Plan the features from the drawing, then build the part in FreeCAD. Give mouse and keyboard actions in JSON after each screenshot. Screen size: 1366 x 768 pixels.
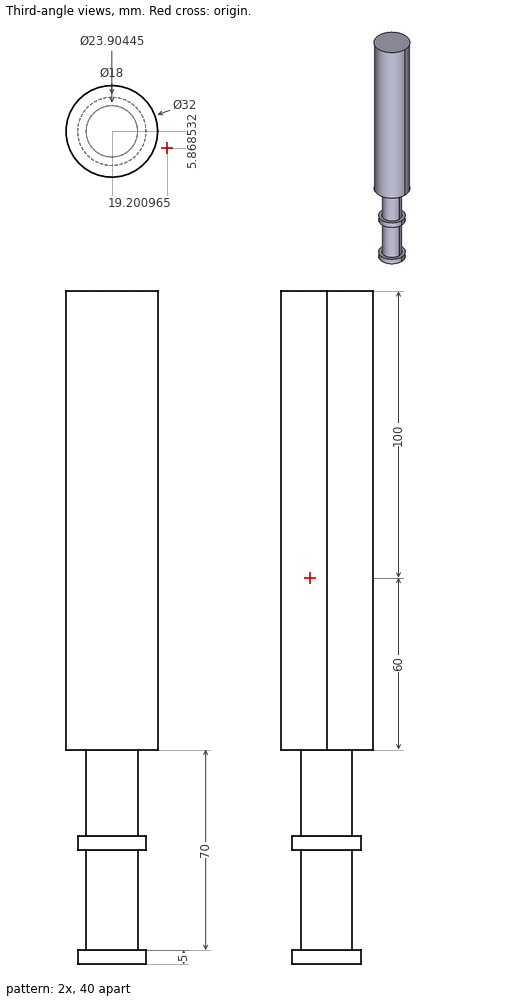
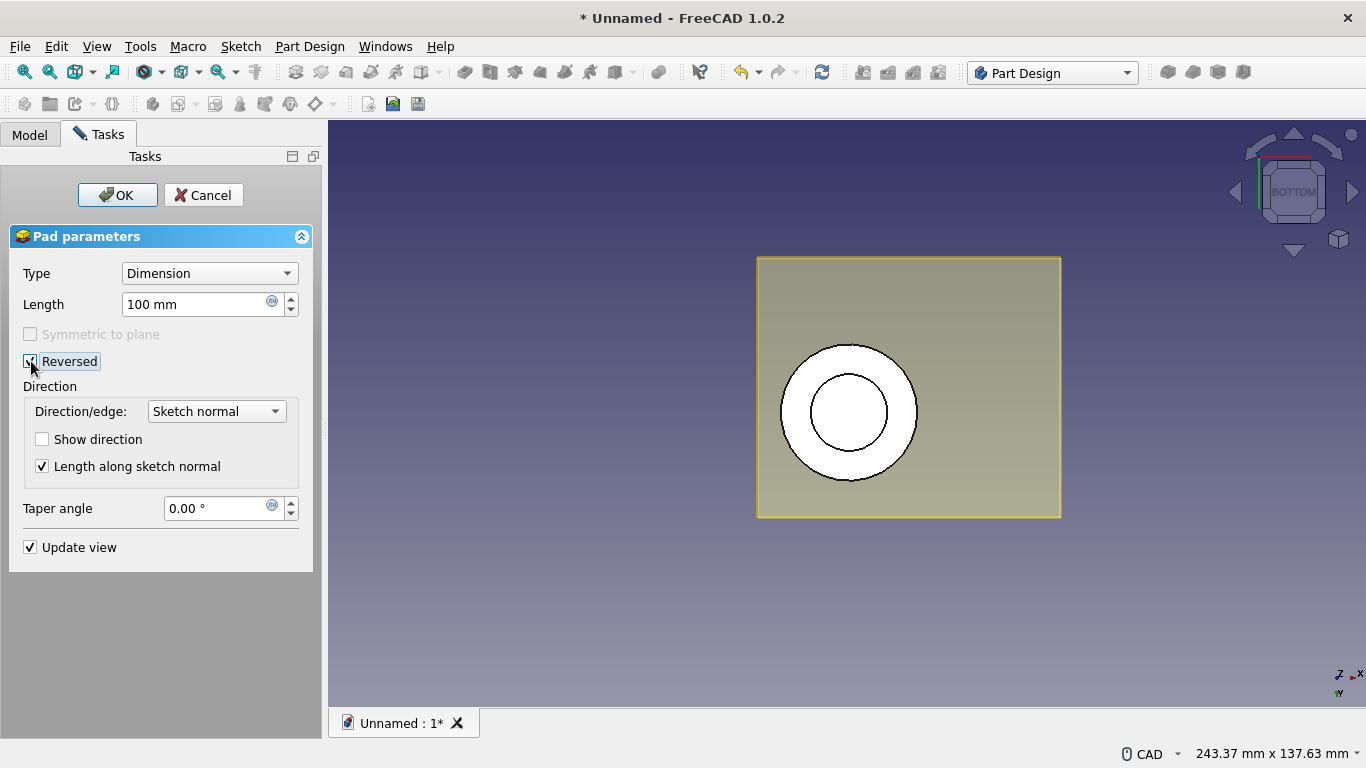
{"action": "left_click", "coordinate": [118, 195]}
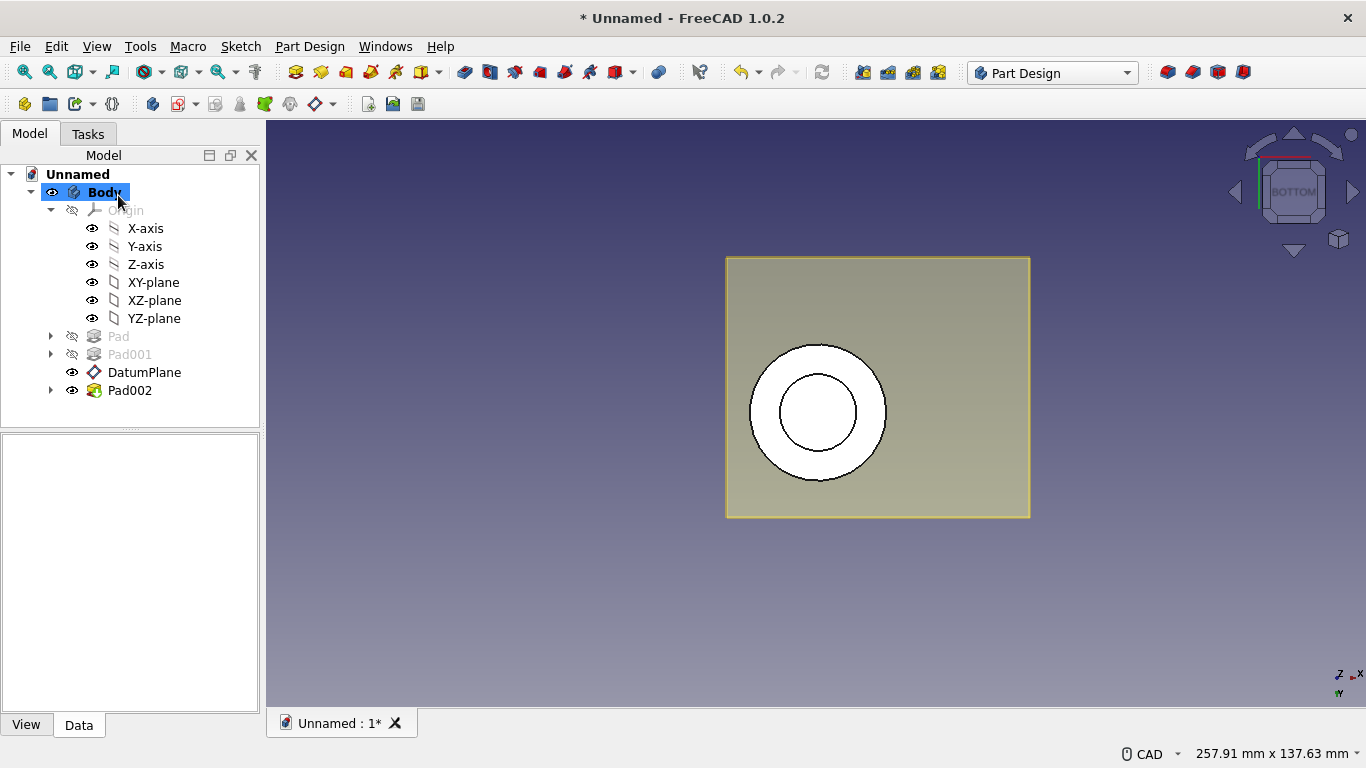
{"action": "left_click", "coordinate": [117, 372]}
{"action": "key", "text": "space"}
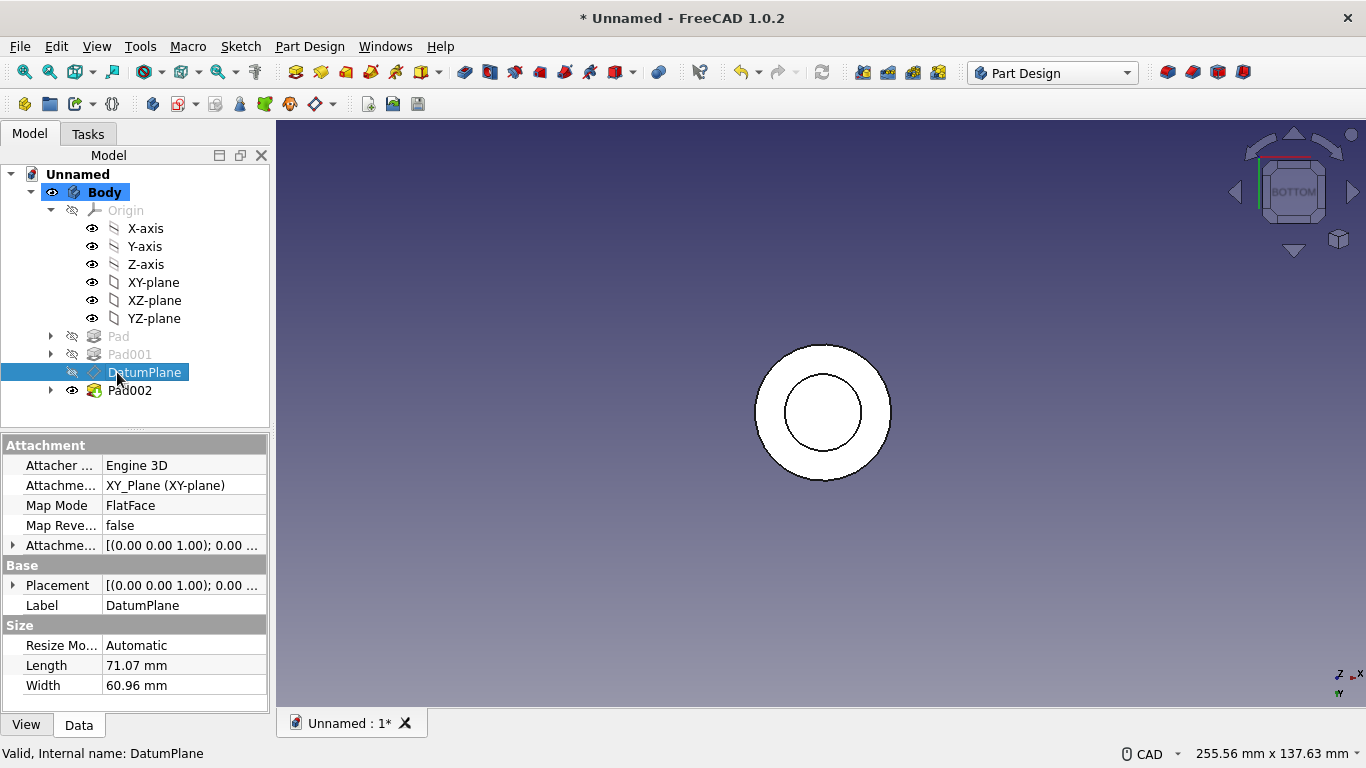
{"action": "key", "text": "v f"}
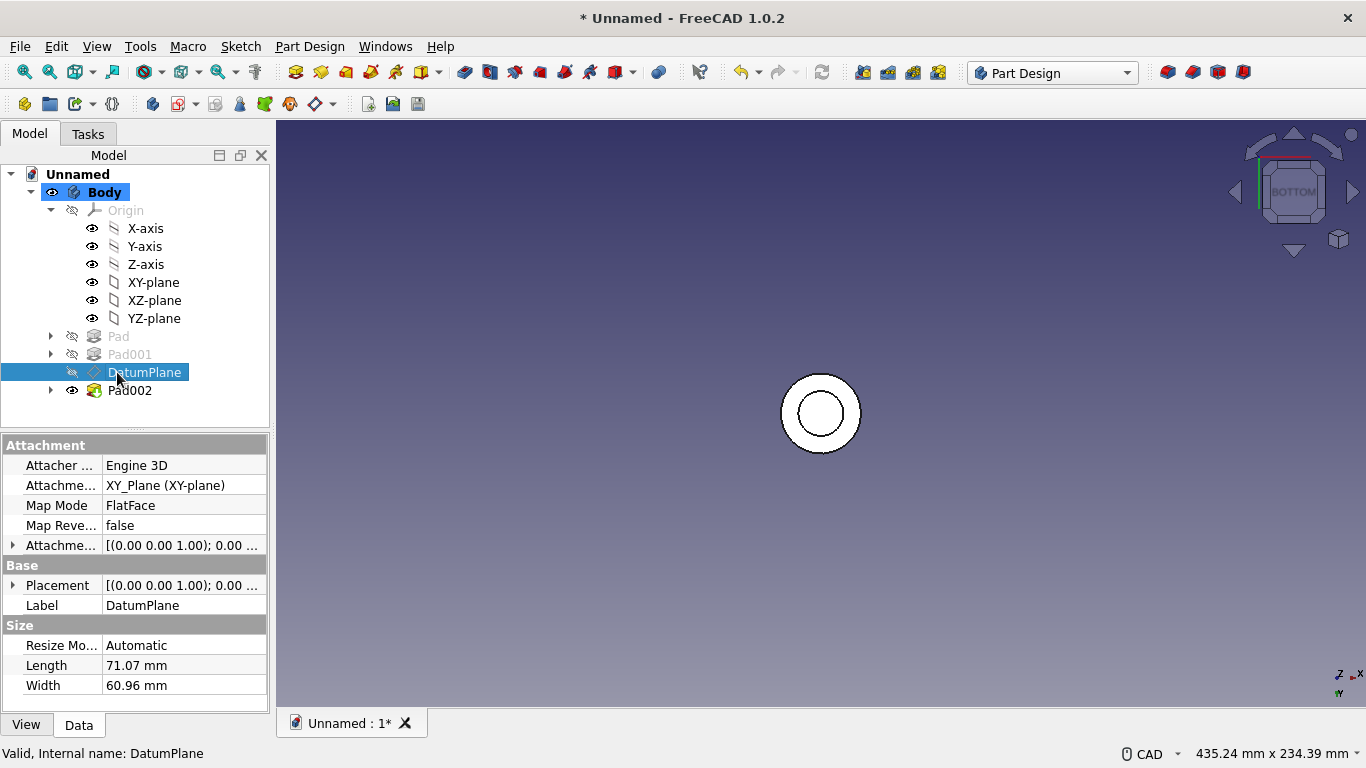
{"action": "left_click", "coordinate": [821, 412]}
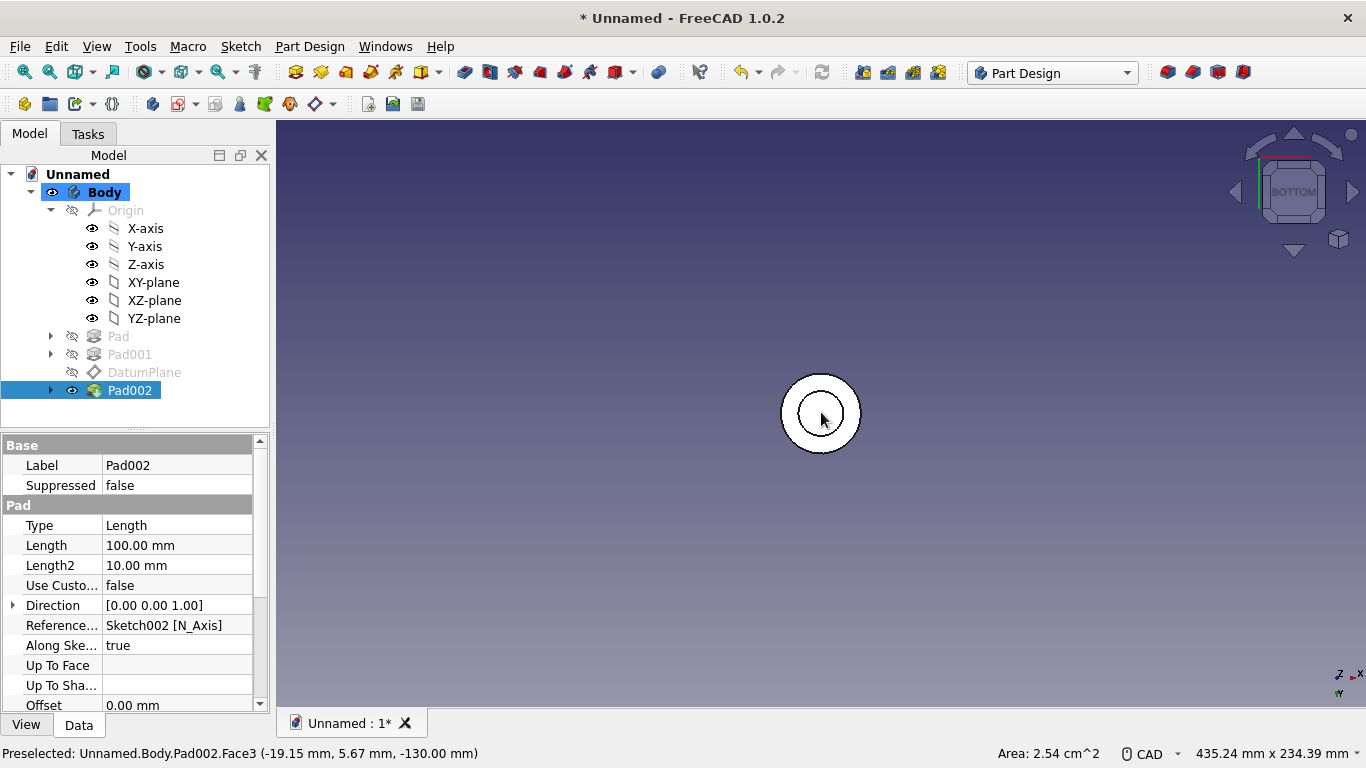
{"action": "left_click", "coordinate": [178, 104]}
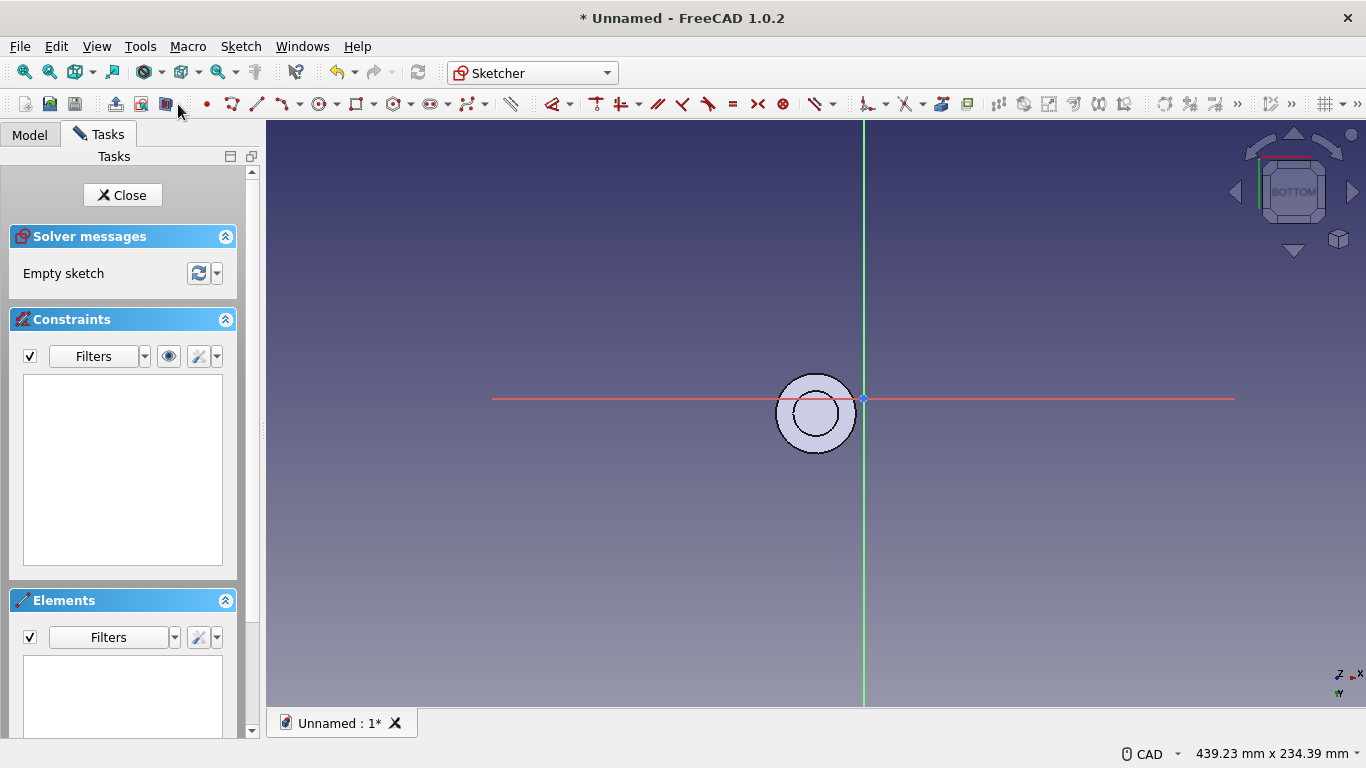
{"action": "scroll", "coordinate": [840, 414], "scroll_direction": "up", "scroll_amount": 9}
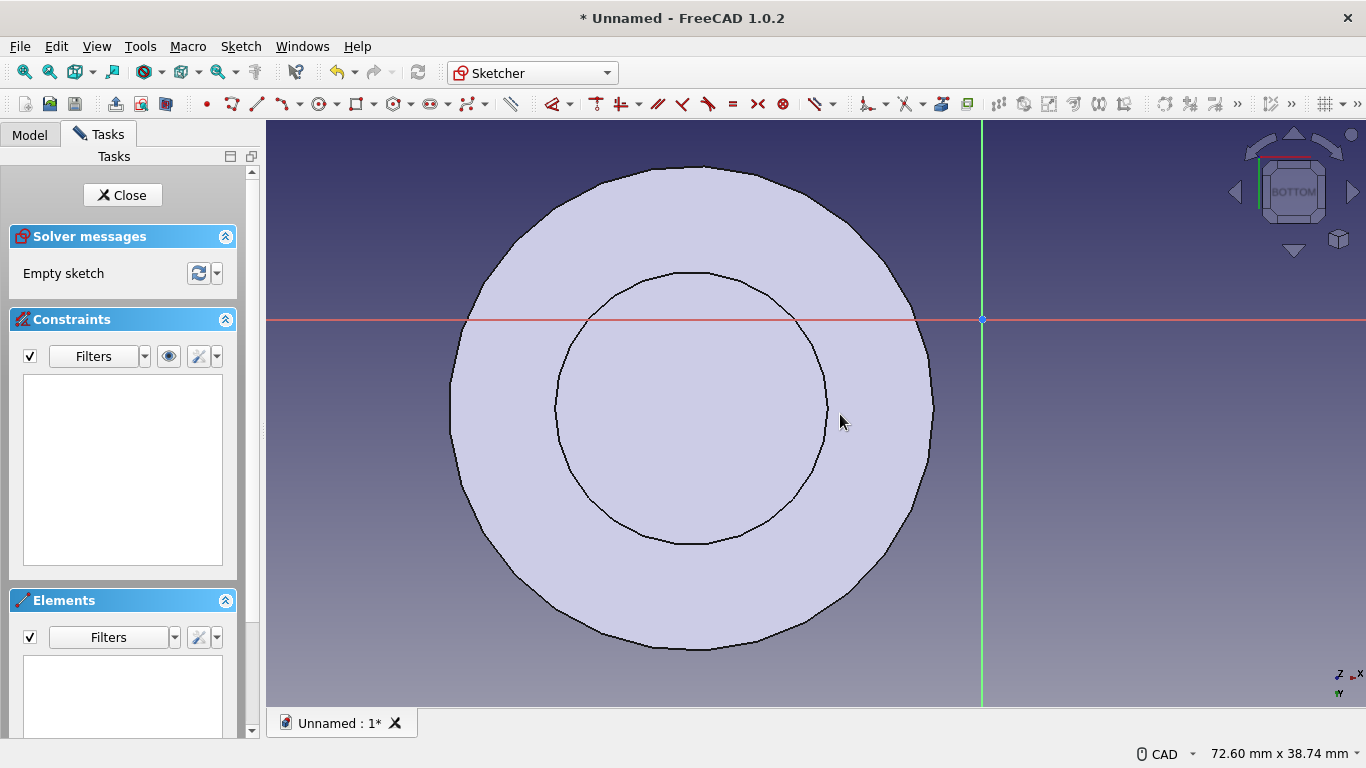
{"action": "key", "text": "g c"}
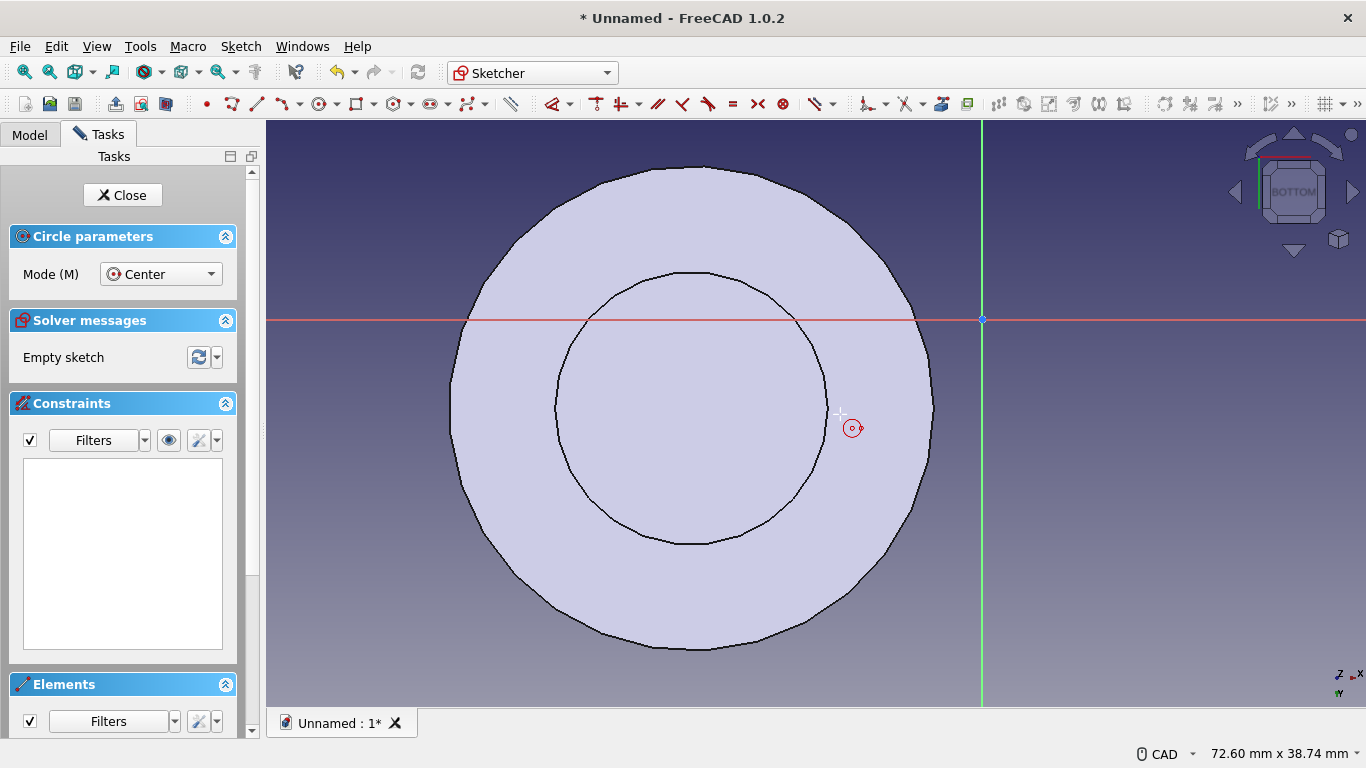
{"action": "left_click", "coordinate": [691, 408]}
{"action": "mouse_move", "coordinate": [820, 280]}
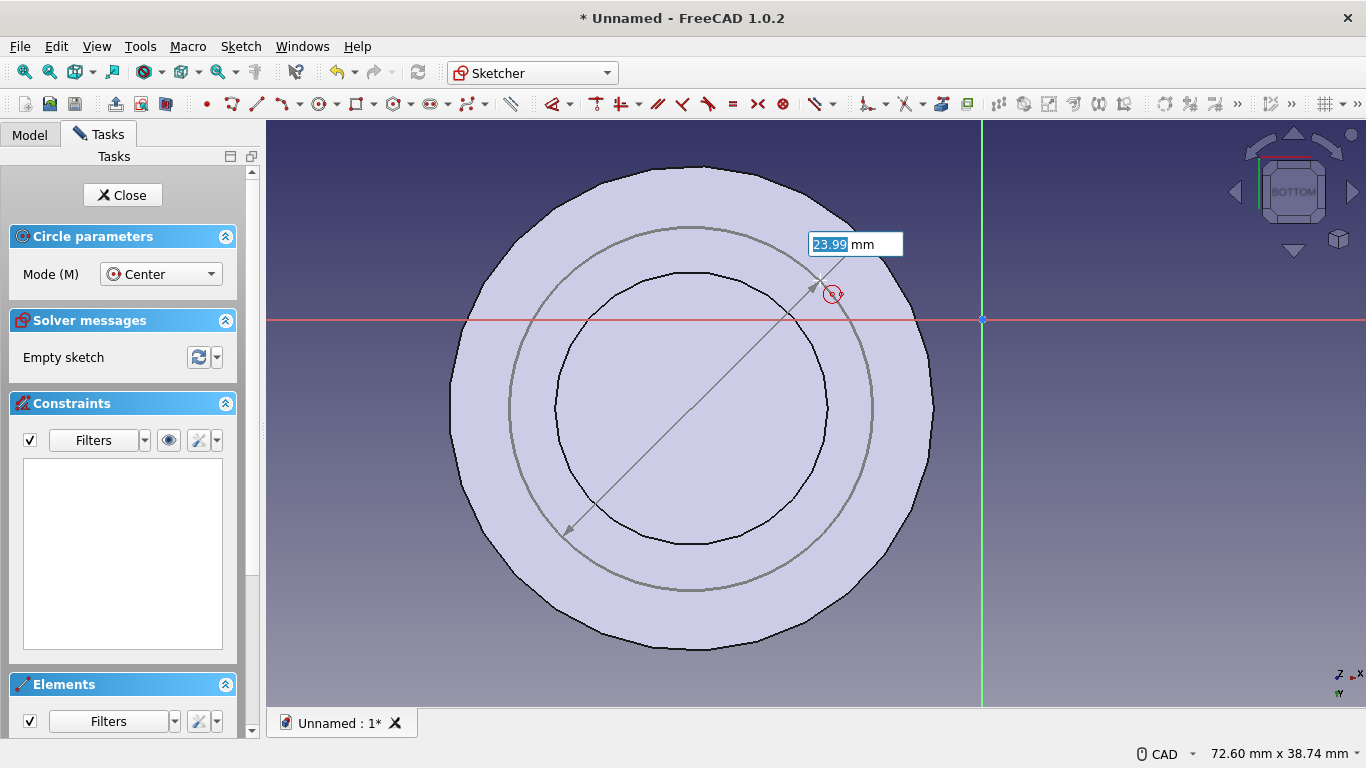
{"action": "type", "text": "23.90445"}
{"action": "key", "text": "Return"}
{"action": "key", "text": "Escape"}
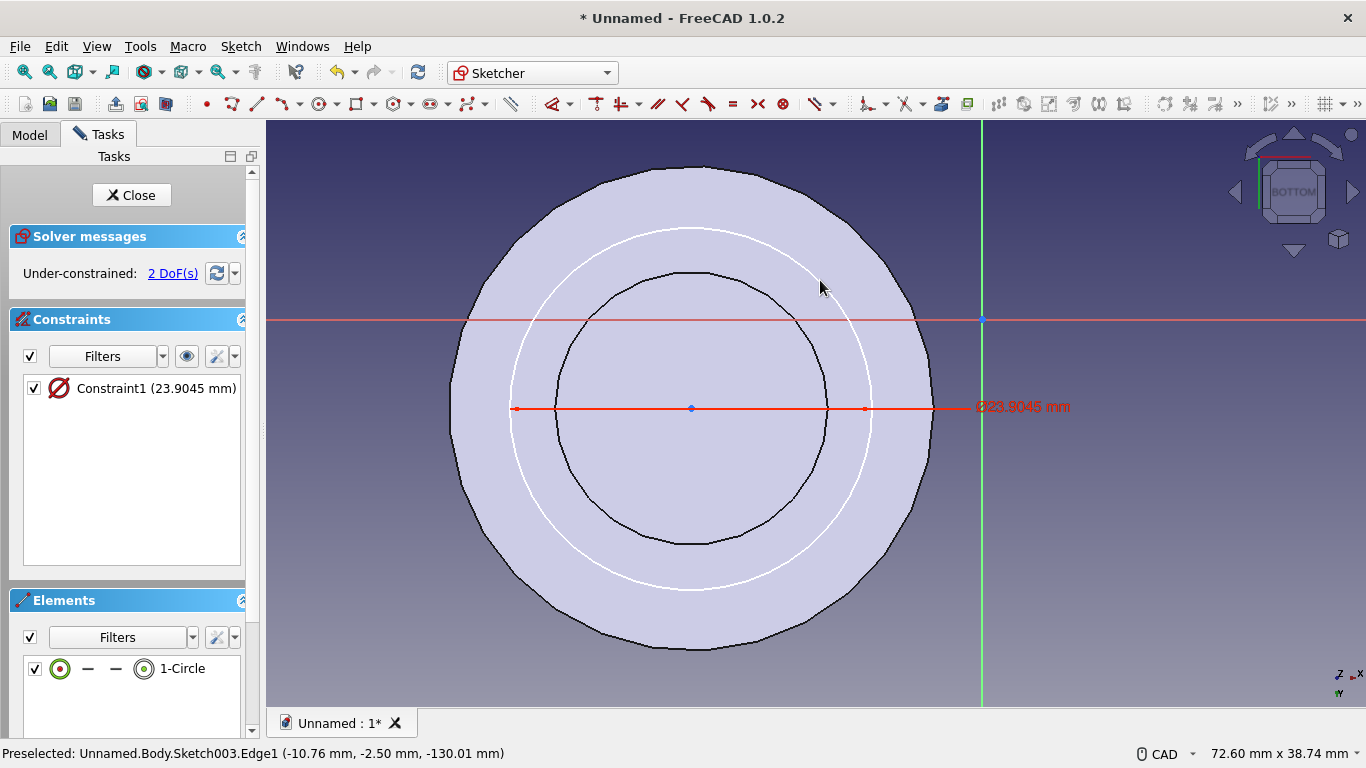
{"action": "left_click", "coordinate": [552, 104]}